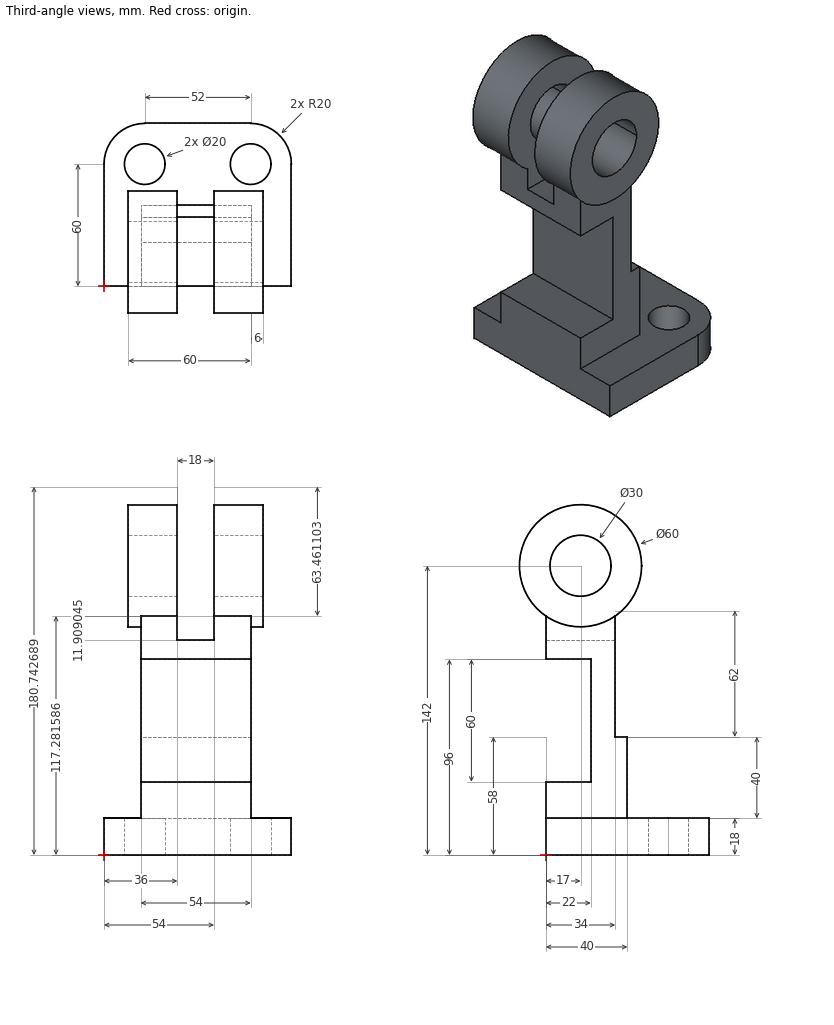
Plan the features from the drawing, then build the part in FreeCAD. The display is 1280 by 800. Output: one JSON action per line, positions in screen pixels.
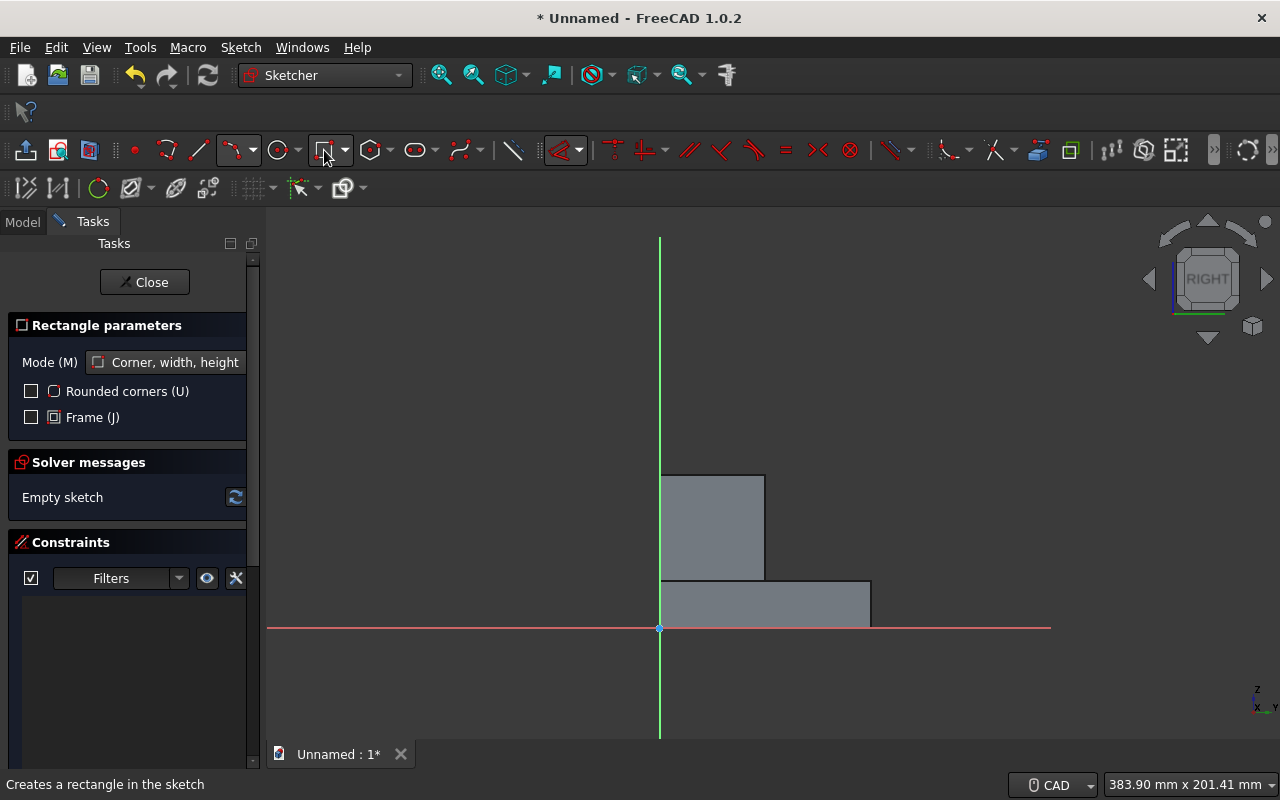
{"action": "left_click", "coordinate": [660, 311]}
{"action": "mouse_move", "coordinate": [749, 475]}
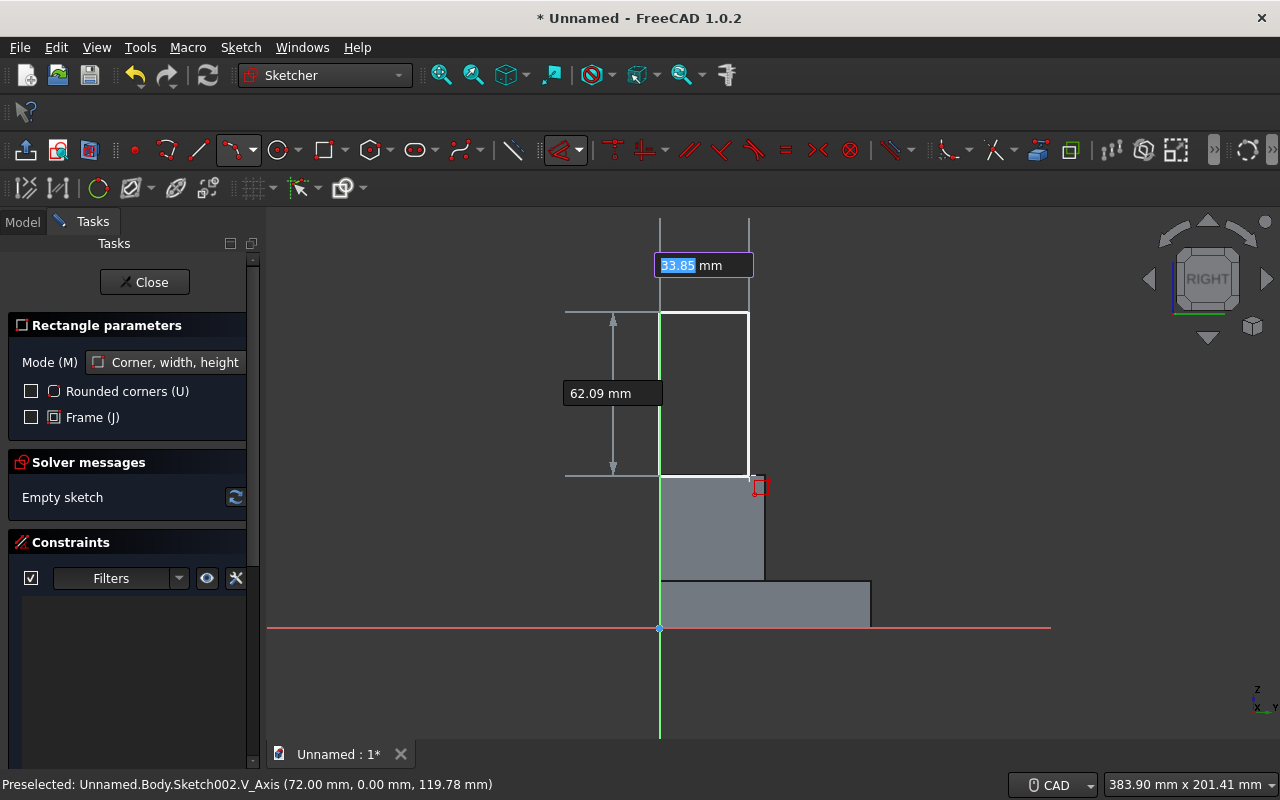
{"action": "type", "text": "34"}
{"action": "key", "text": "Tab"}
{"action": "type", "text": "62"}
{"action": "key", "text": "Return"}
{"action": "key", "text": "Escape"}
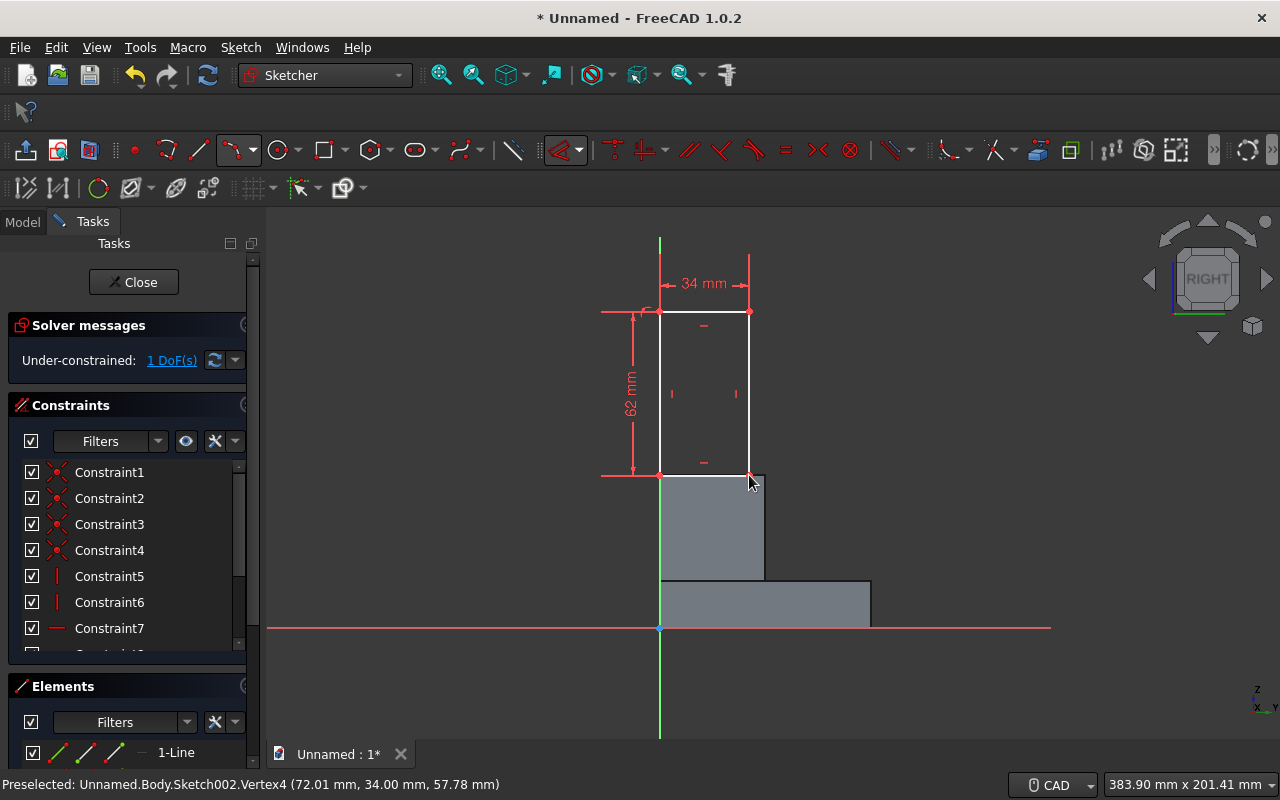
{"action": "left_click", "coordinate": [660, 476]}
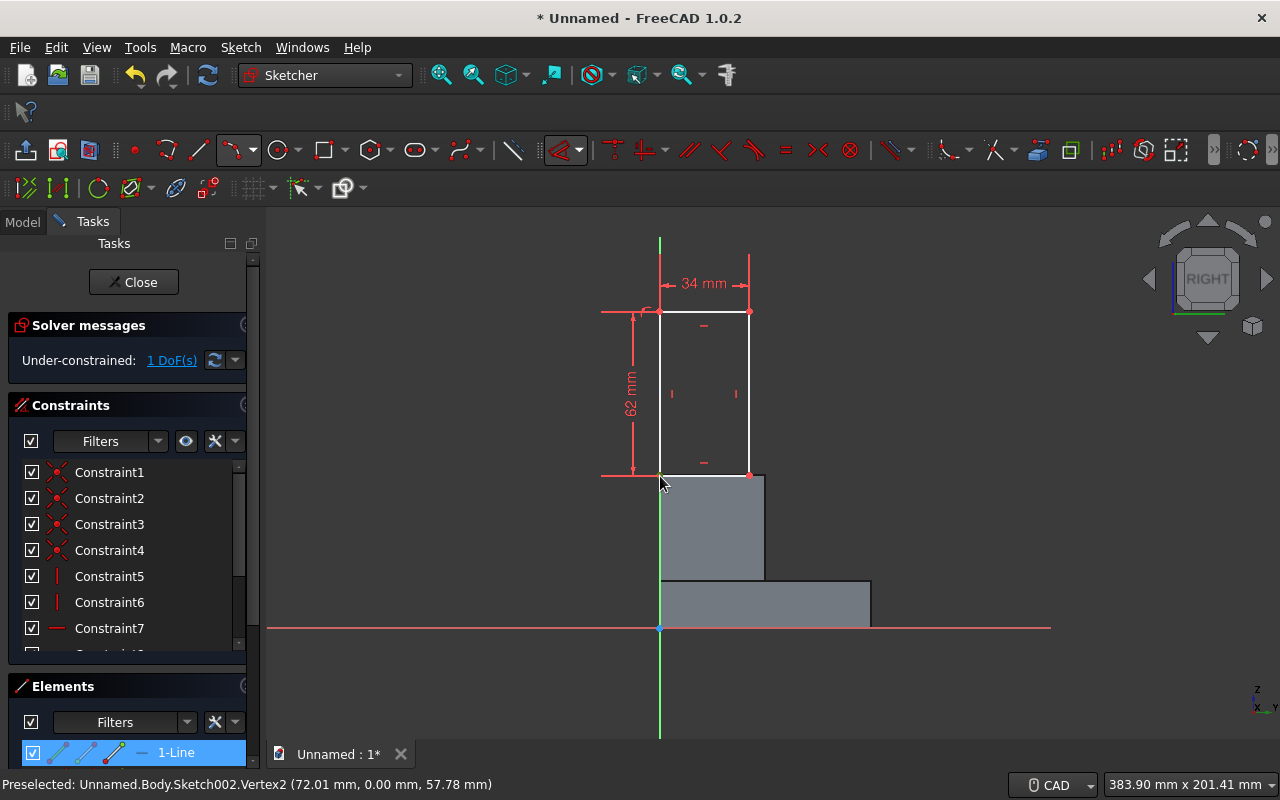
{"action": "left_click", "coordinate": [582, 150]}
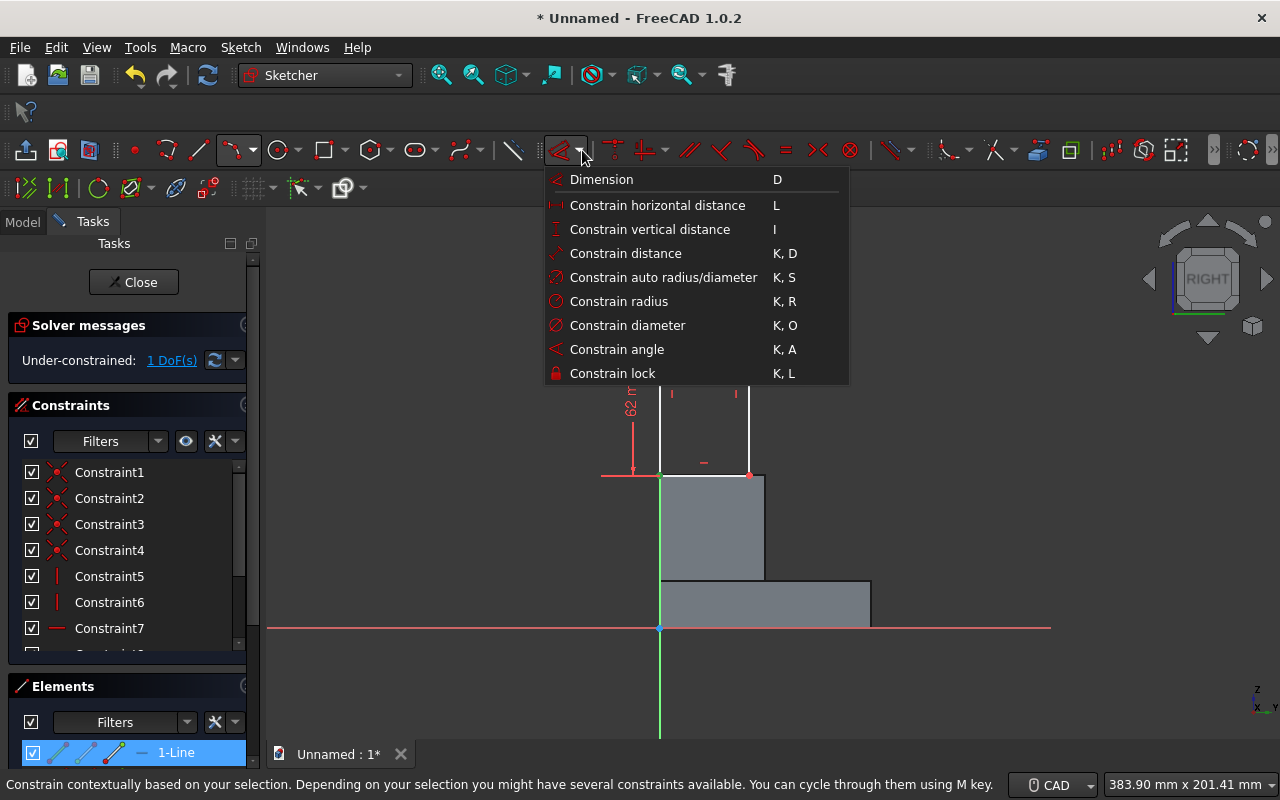
{"action": "left_click", "coordinate": [697, 229]}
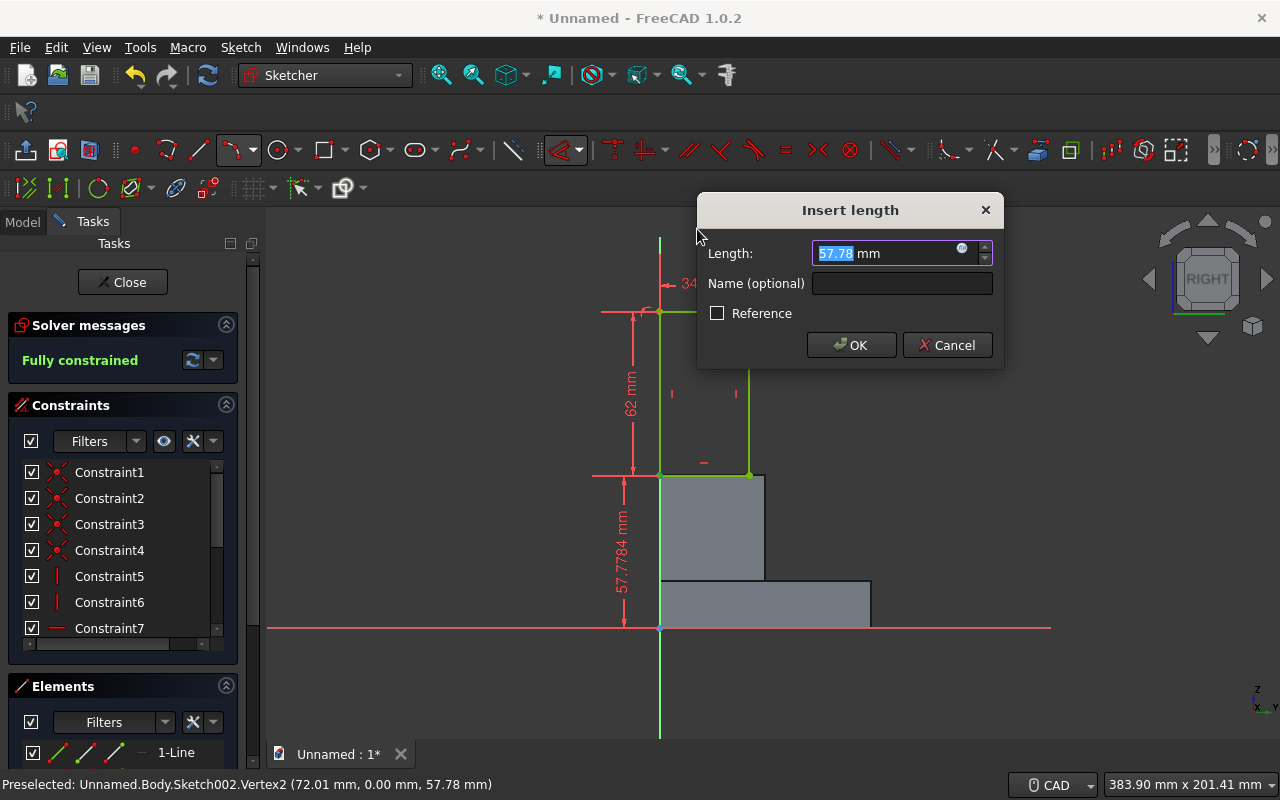
{"action": "type", "text": "58"}
{"action": "key", "text": "Return"}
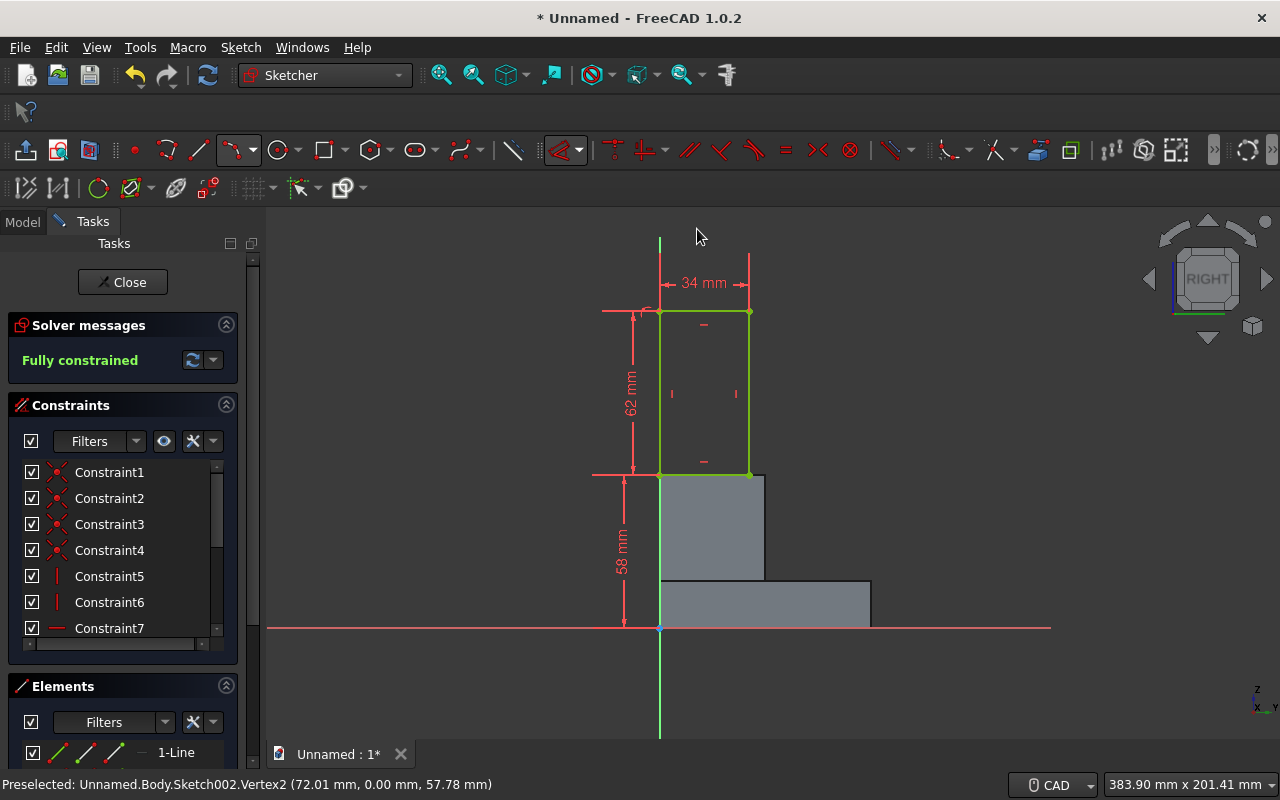
{"action": "left_click", "coordinate": [123, 282]}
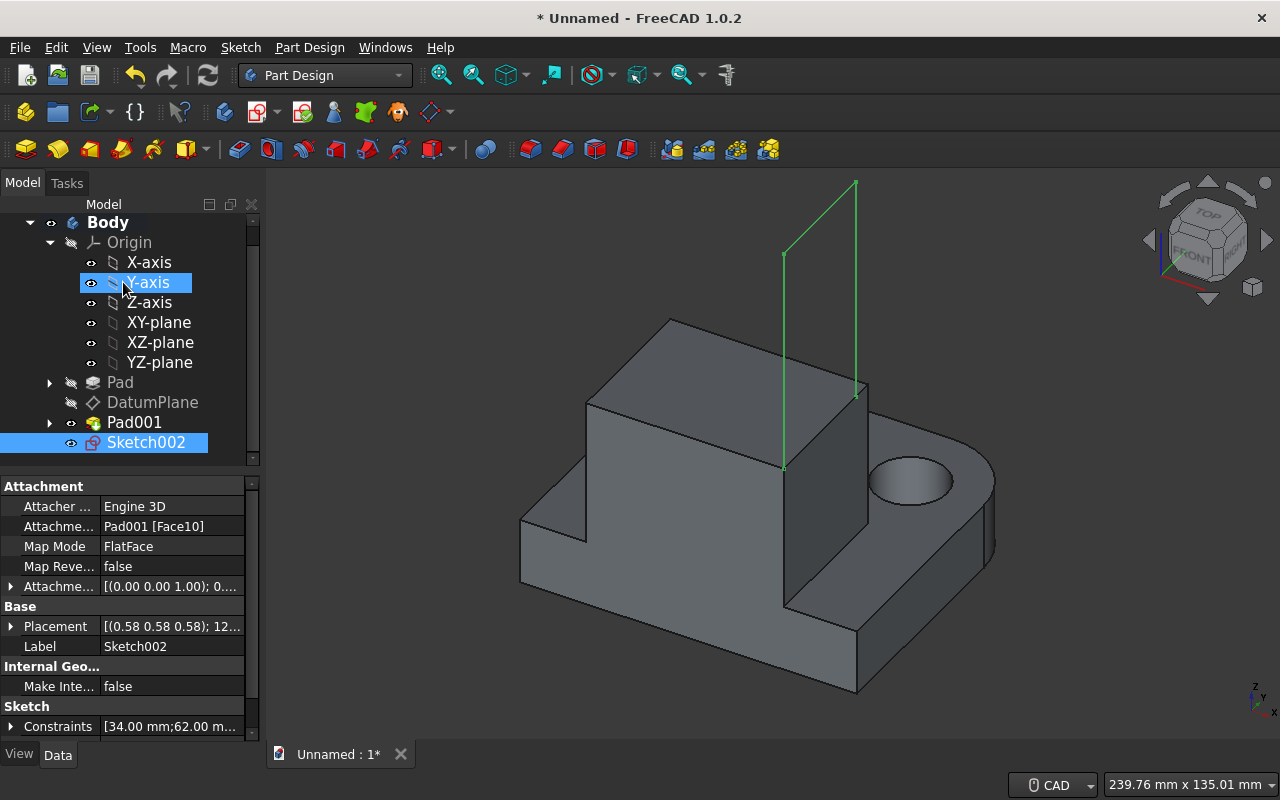
{"action": "left_click", "coordinate": [26, 150]}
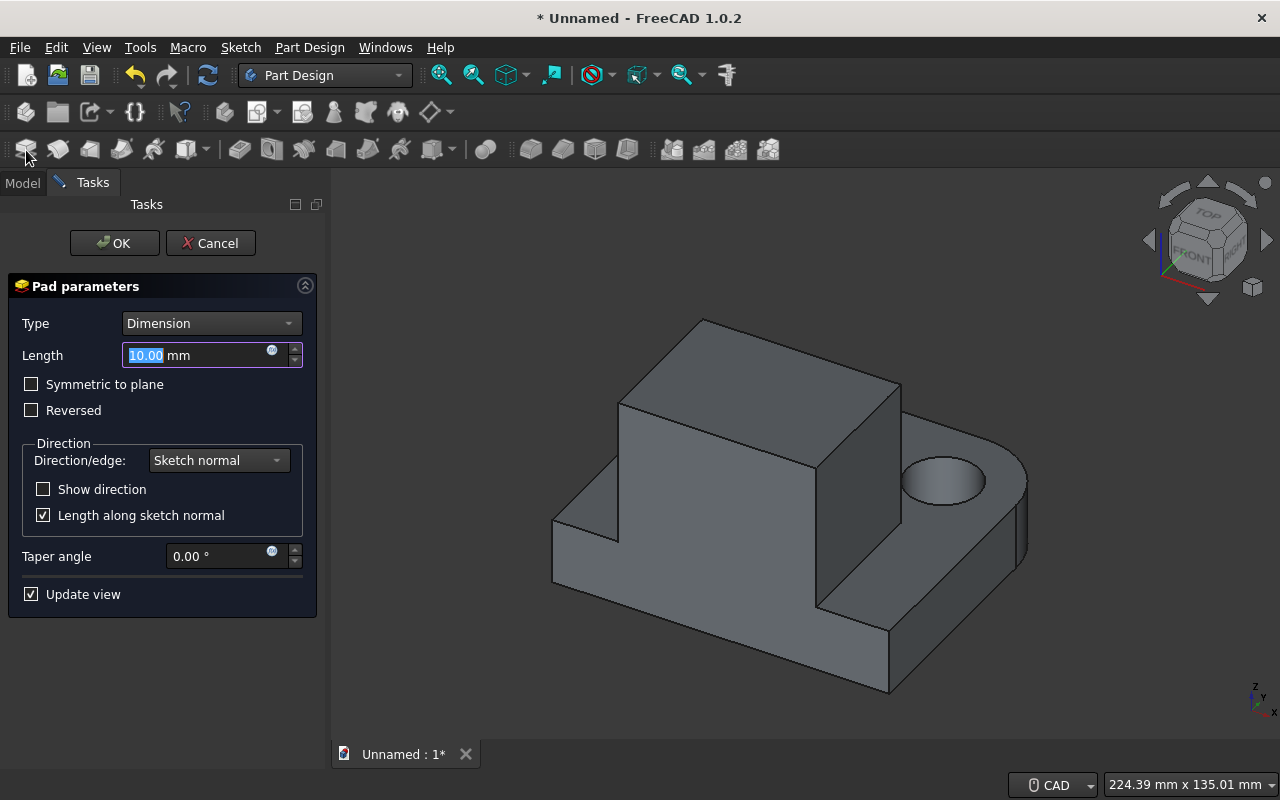
{"action": "type", "text": "54"}
{"action": "key", "text": "Tab"}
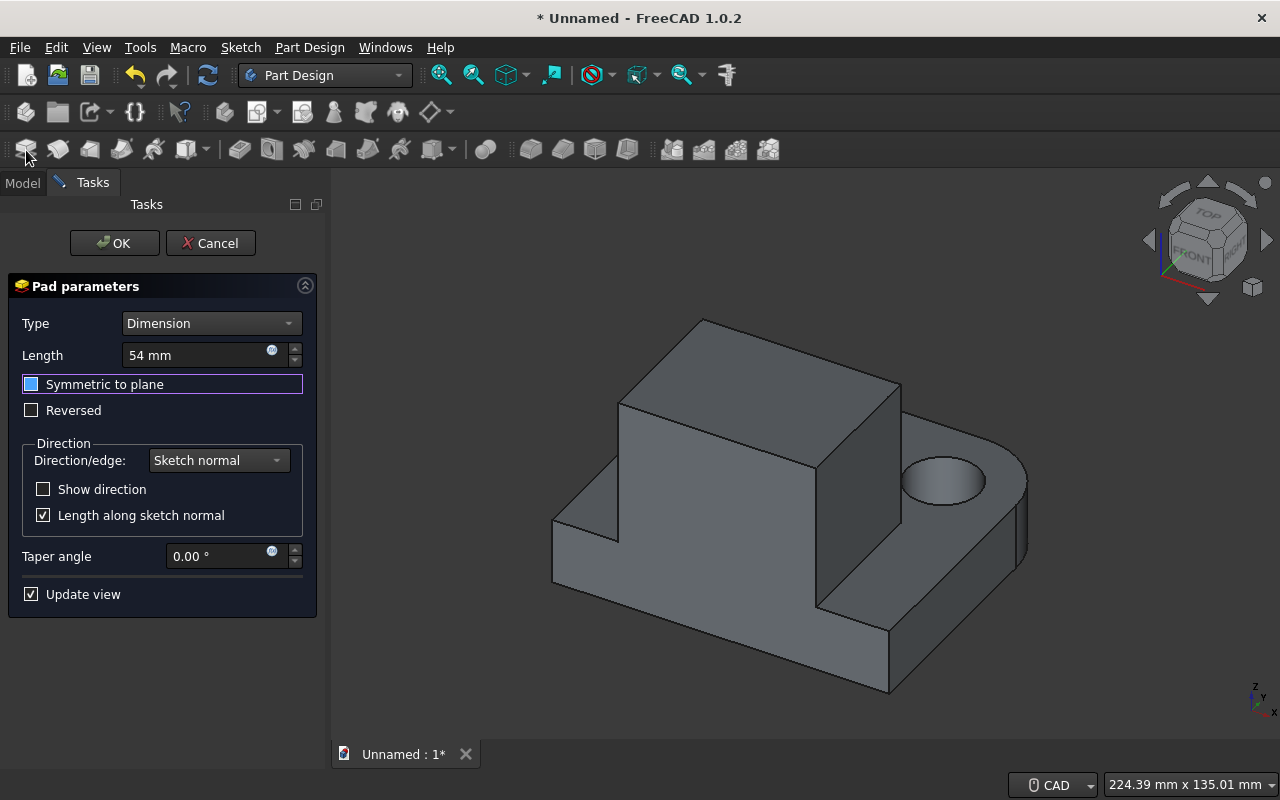
{"action": "left_click", "coordinate": [30, 410]}